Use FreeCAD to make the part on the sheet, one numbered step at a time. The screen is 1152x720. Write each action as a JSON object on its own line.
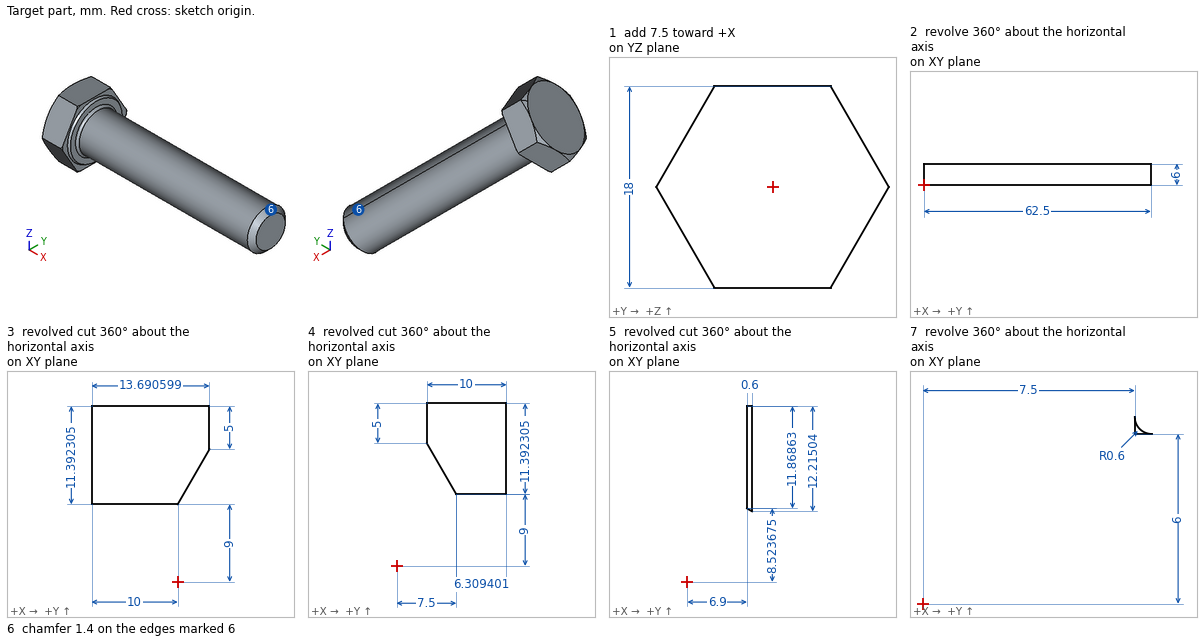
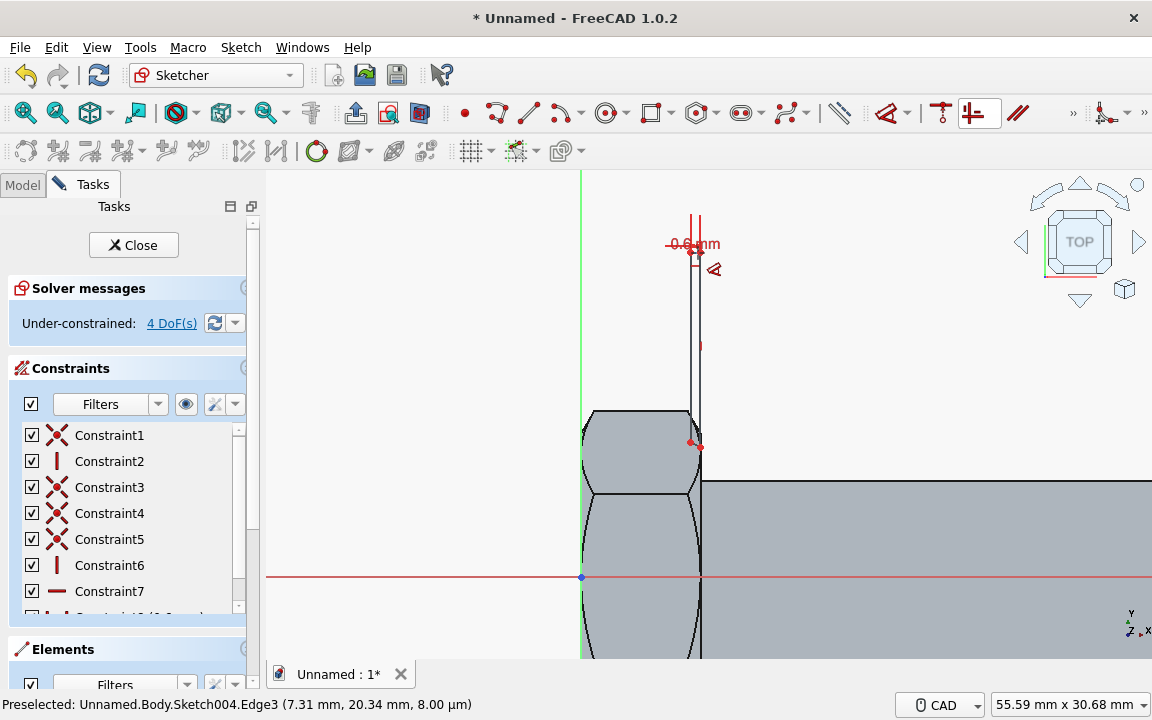
{"action": "left_click", "coordinate": [691, 442]}
{"action": "left_click", "coordinate": [636, 611]}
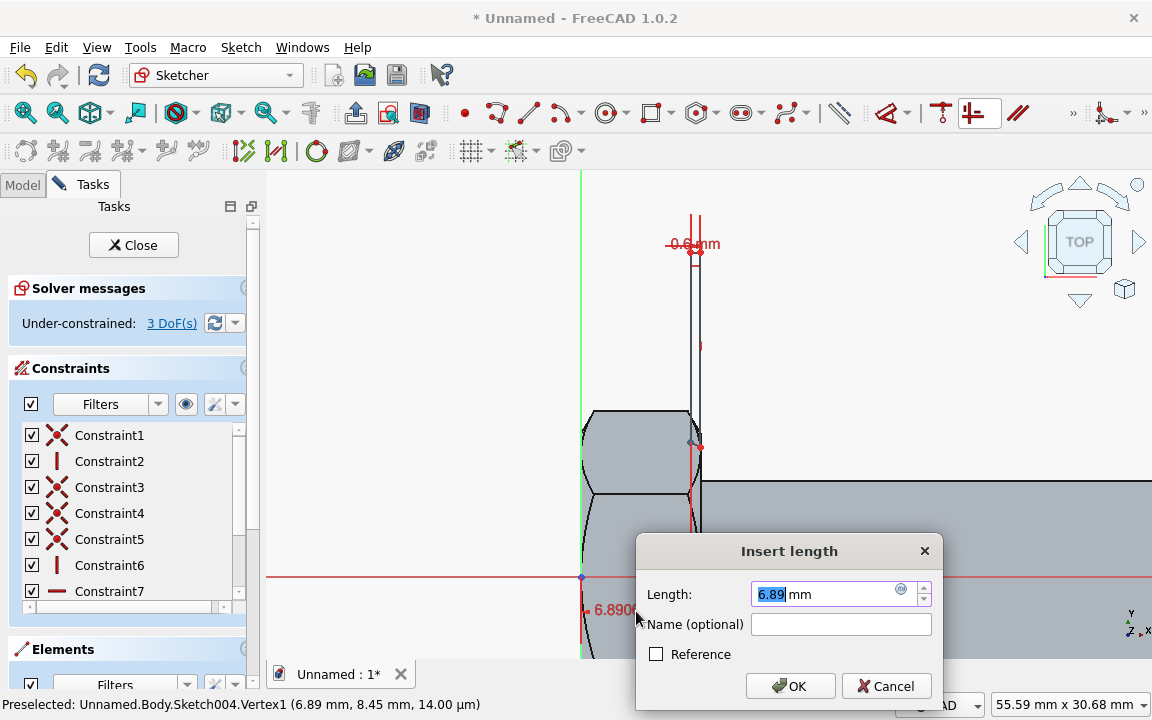
{"action": "type", "text": "6.9"}
{"action": "key", "text": "Return"}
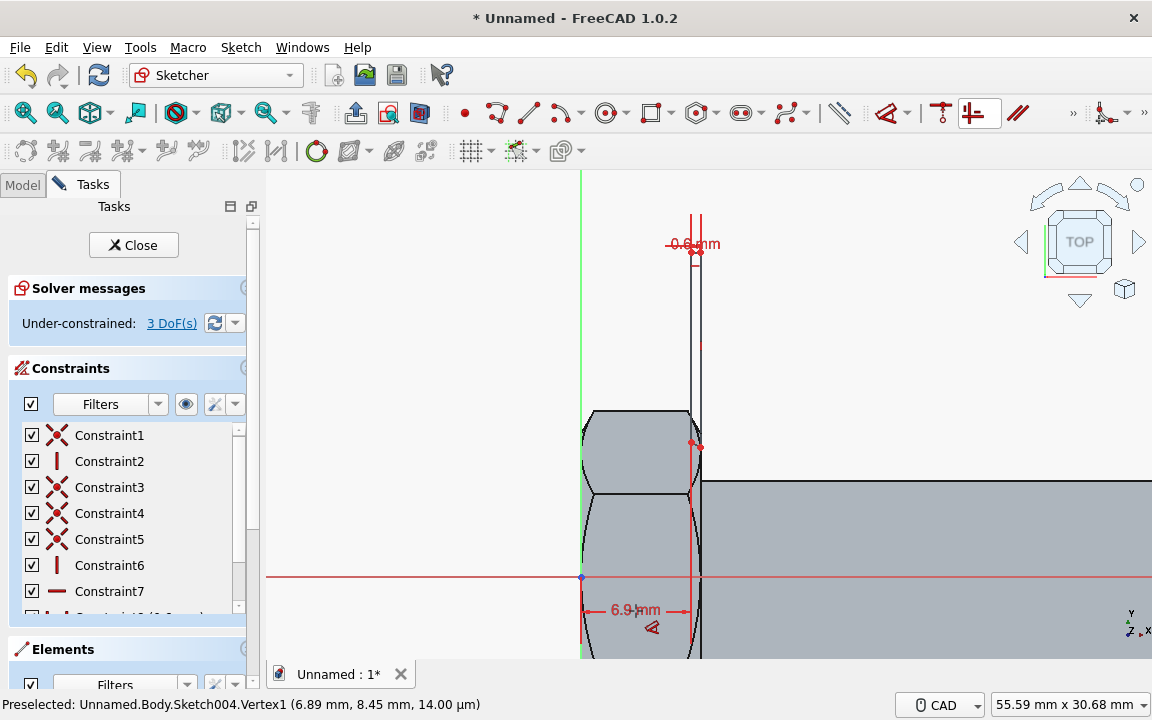
{"action": "scroll", "coordinate": [701, 389], "scroll_direction": "up", "scroll_amount": 2}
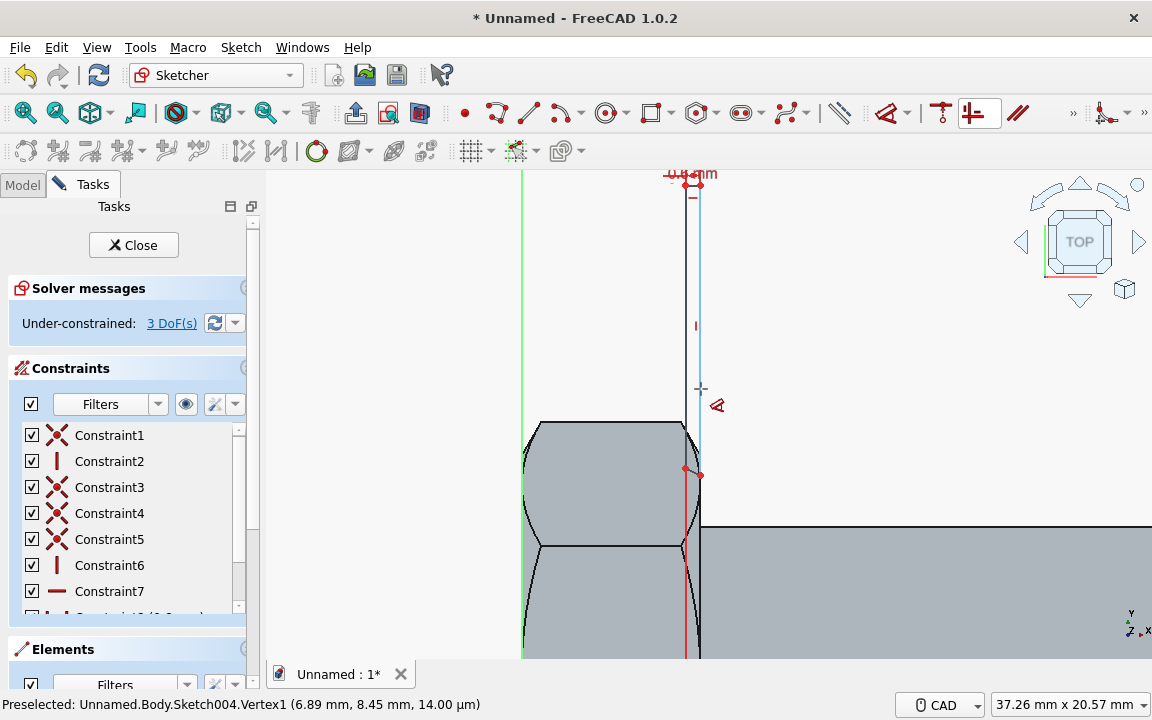
{"action": "left_click", "coordinate": [700, 389]}
{"action": "left_click", "coordinate": [734, 337]}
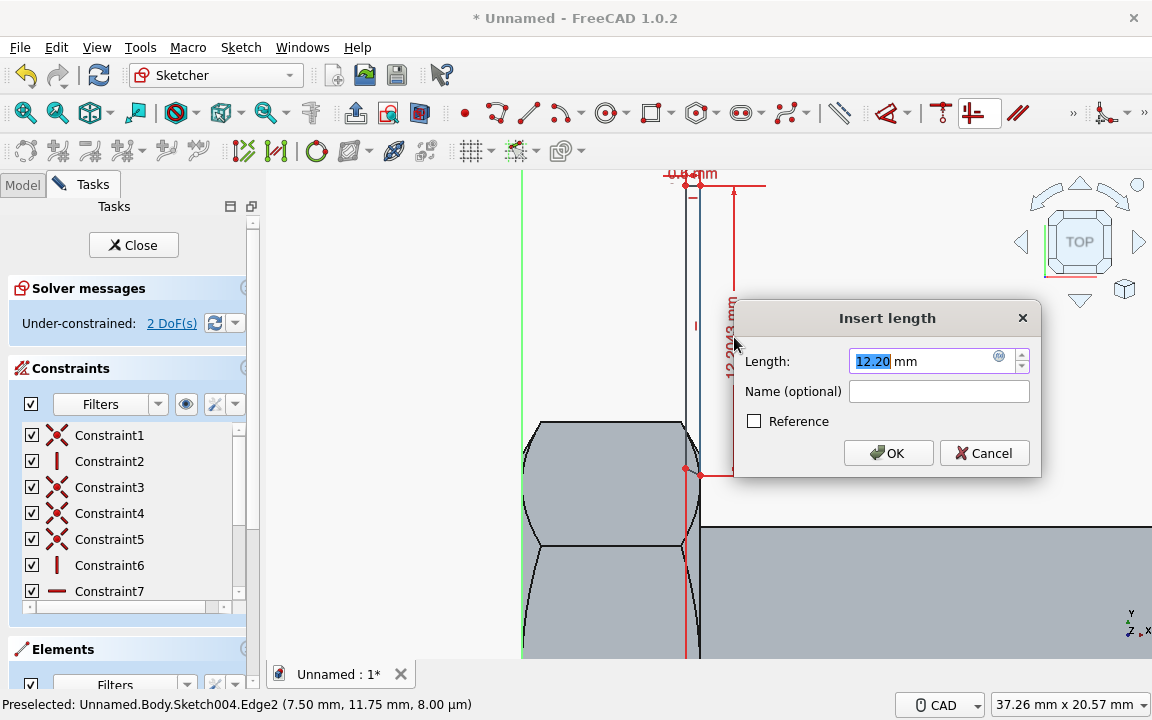
{"action": "type", "text": "12.21504"}
{"action": "key", "text": "Return"}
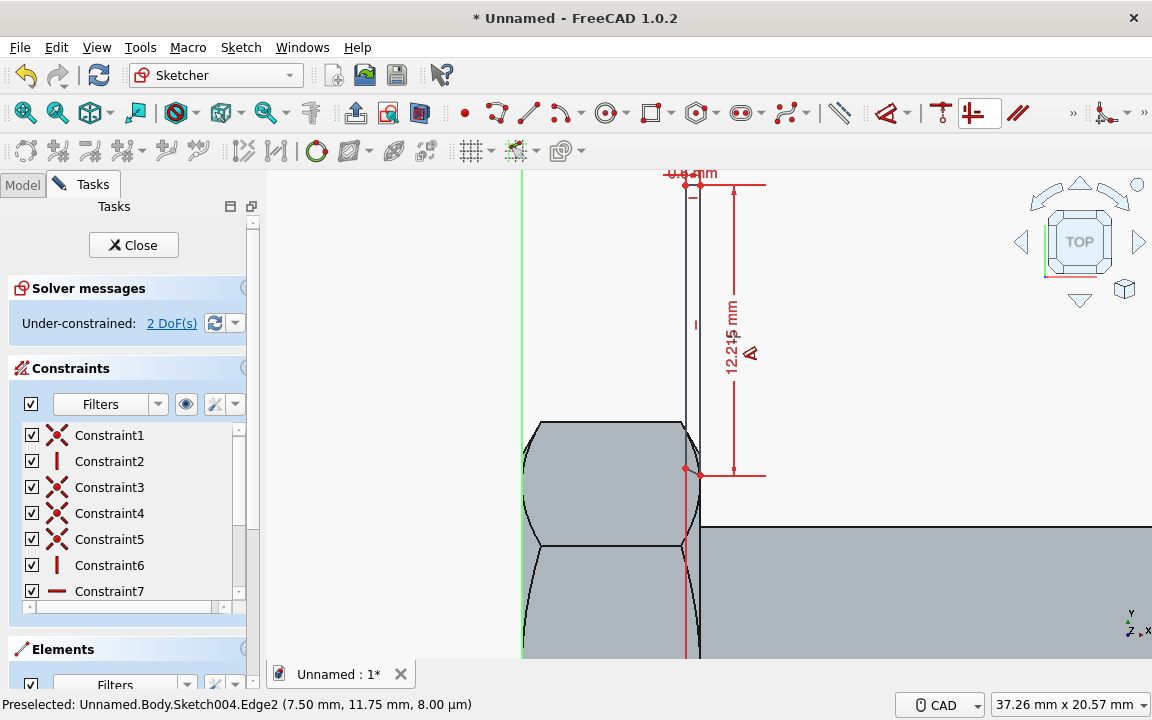
{"action": "left_click", "coordinate": [686, 270]}
{"action": "left_click", "coordinate": [720, 271]}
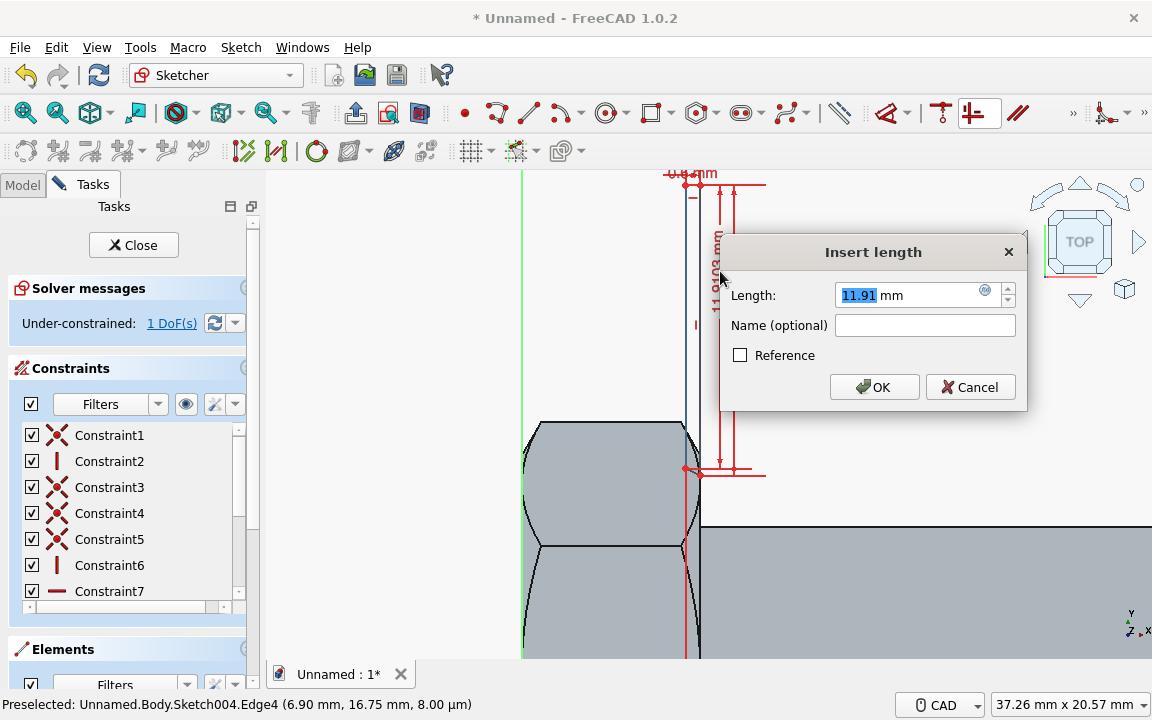
{"action": "type", "text": "11.86863"}
{"action": "key", "text": "Return"}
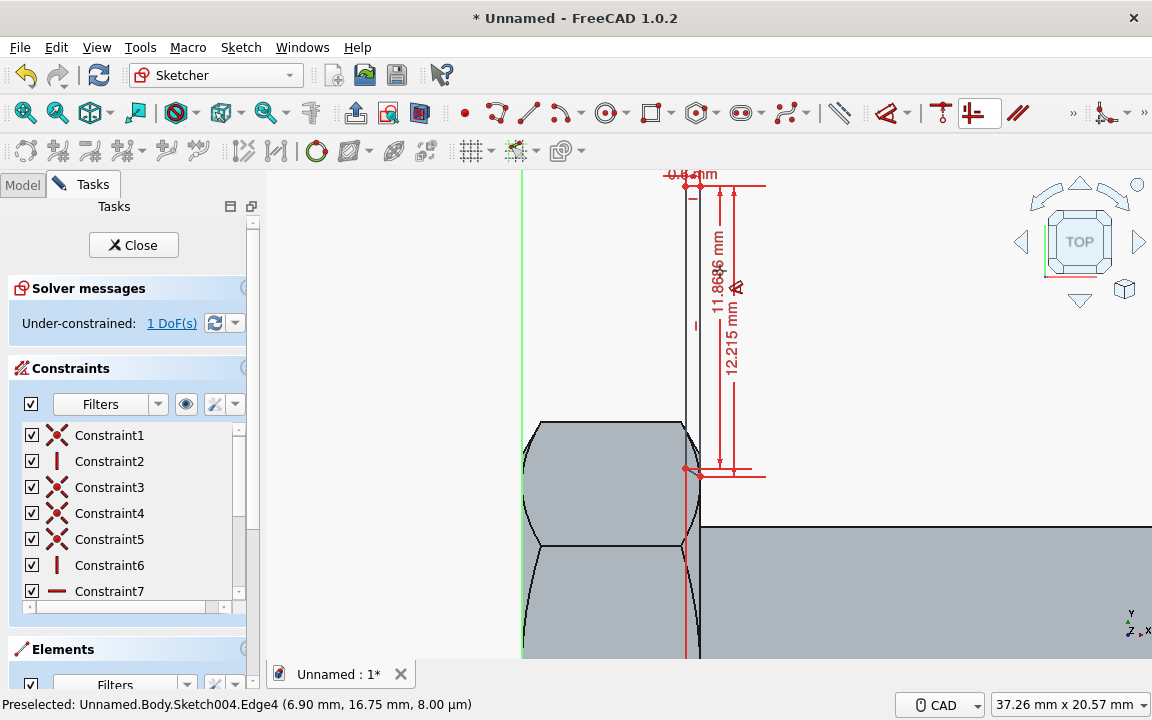
{"action": "left_click", "coordinate": [686, 469]}
{"action": "left_click", "coordinate": [488, 550]}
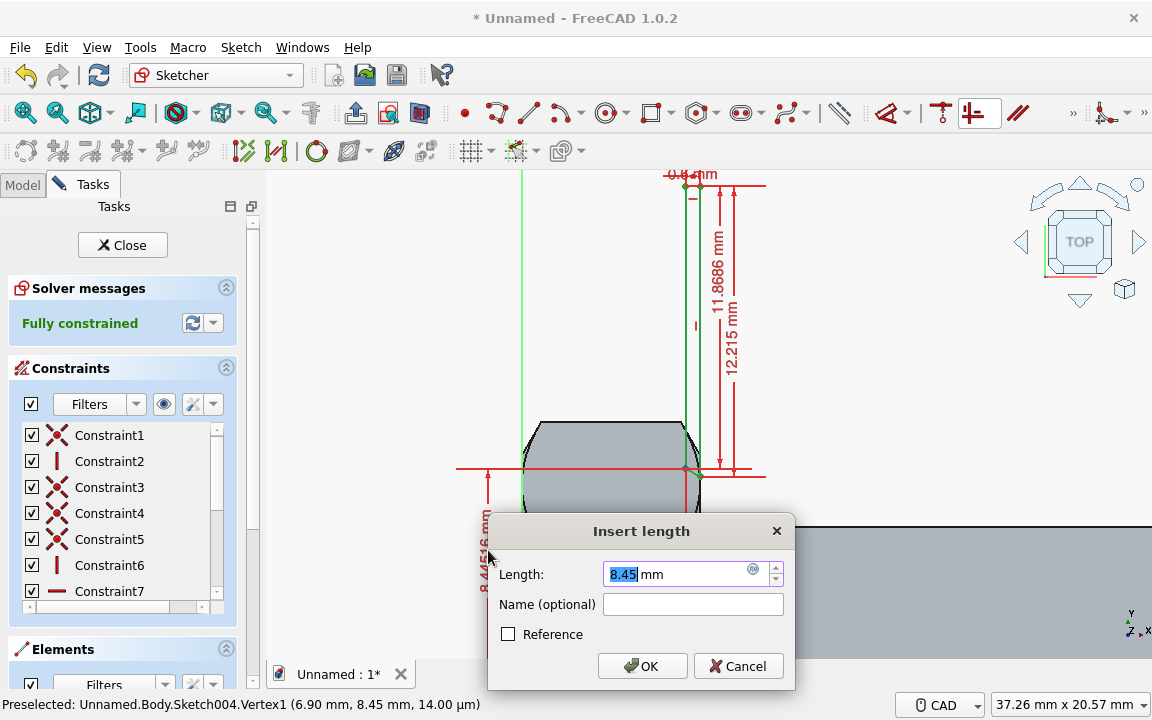
{"action": "type", "text": "8.523675"}
{"action": "key", "text": "Return"}
{"action": "key", "text": "Escape"}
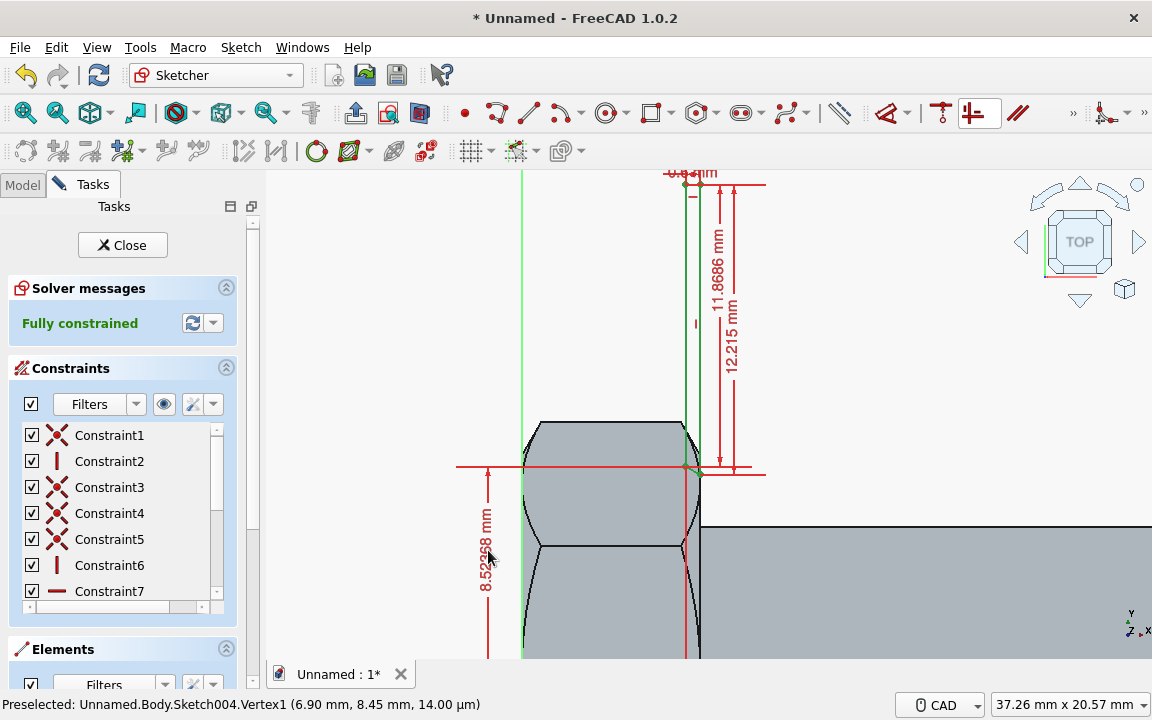
{"action": "left_click", "coordinate": [123, 245]}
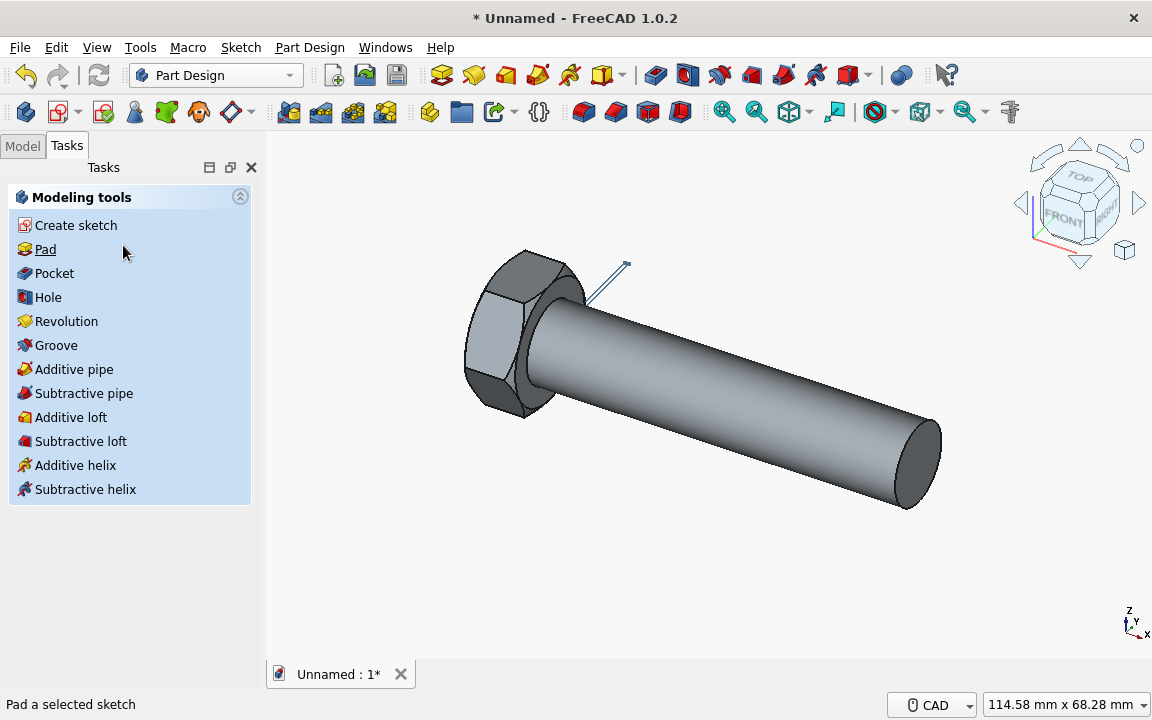
{"action": "left_click", "coordinate": [720, 76]}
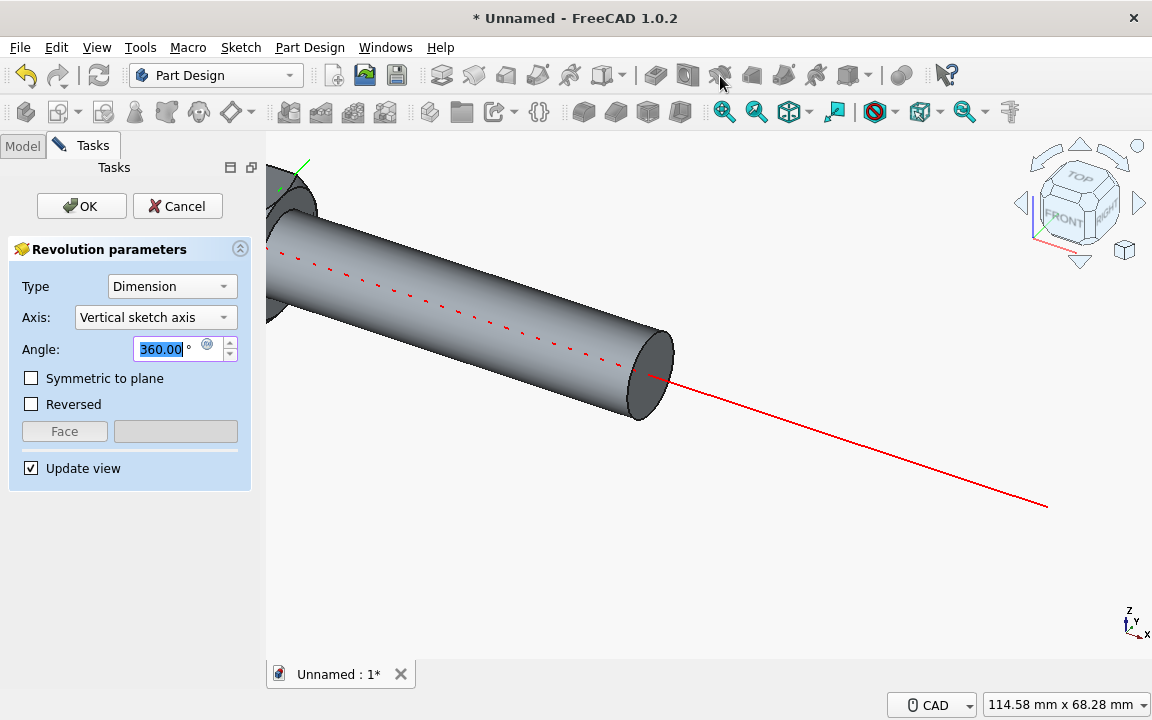
{"action": "left_click", "coordinate": [156, 318]}